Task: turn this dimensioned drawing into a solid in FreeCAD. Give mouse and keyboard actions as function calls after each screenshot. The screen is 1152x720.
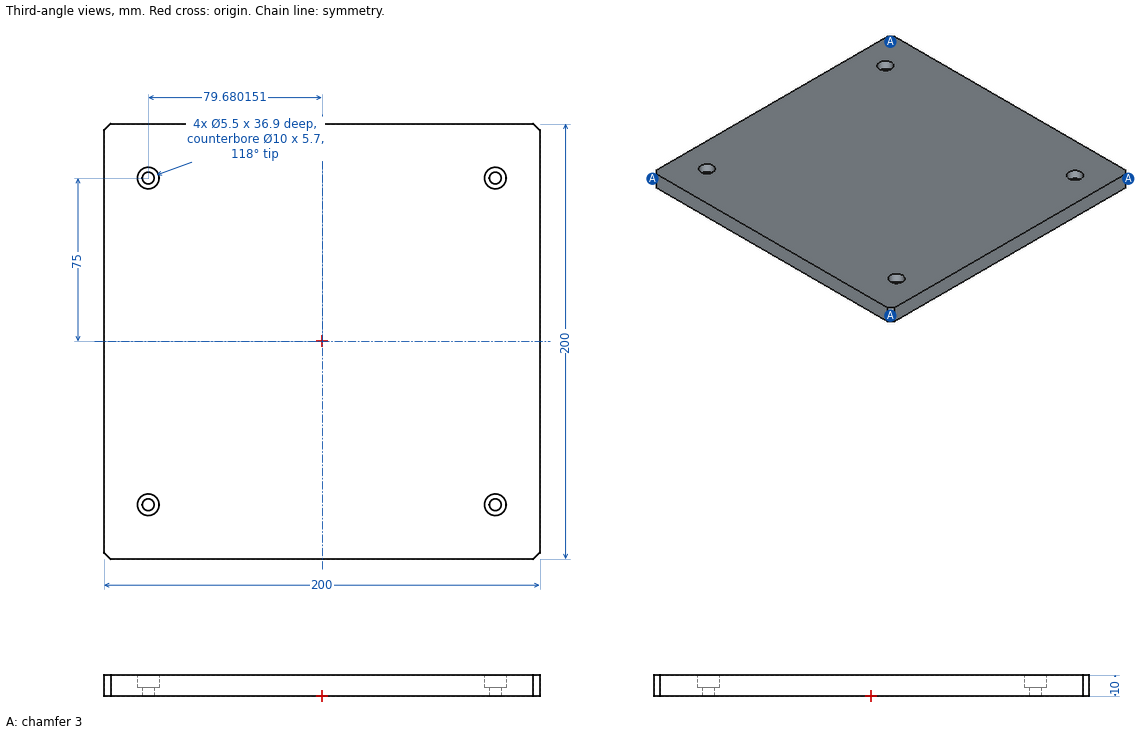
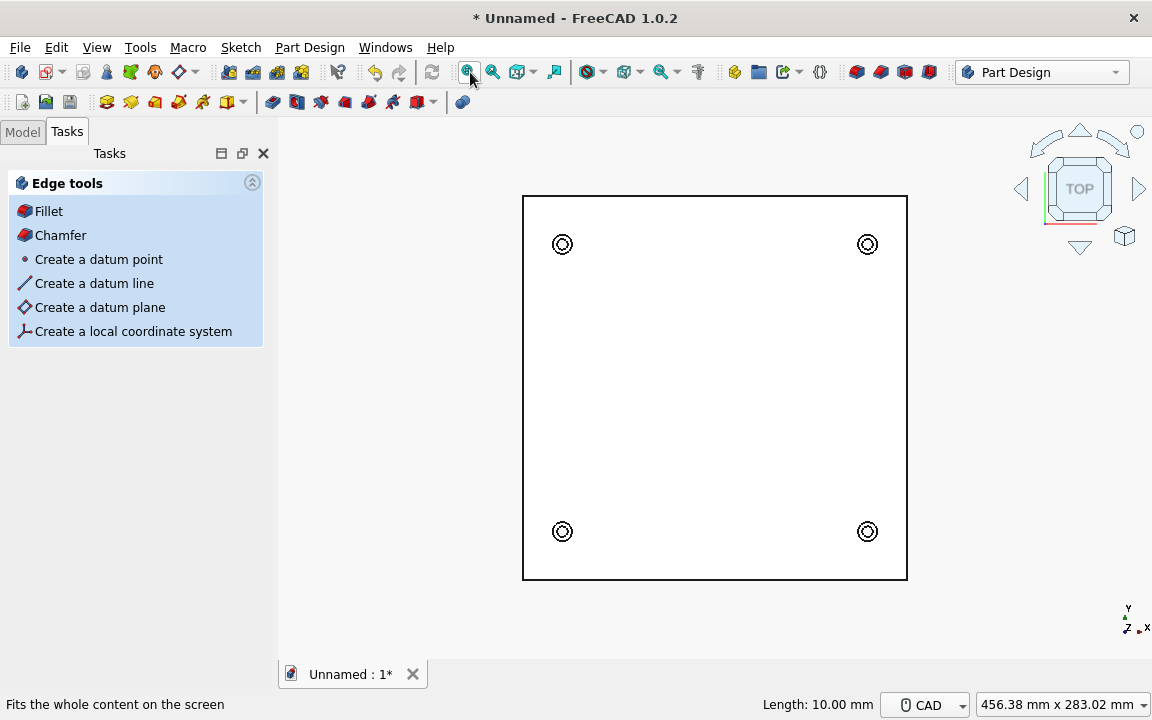
scroll(523, 579, up, 4)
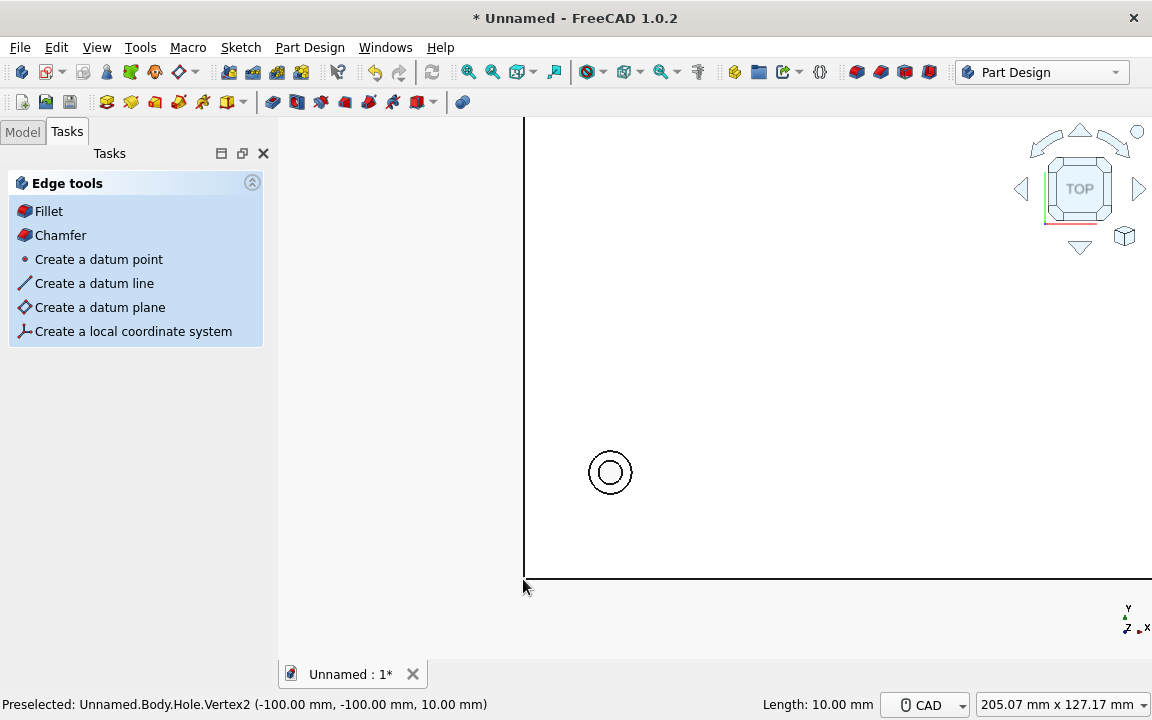
click(470, 72)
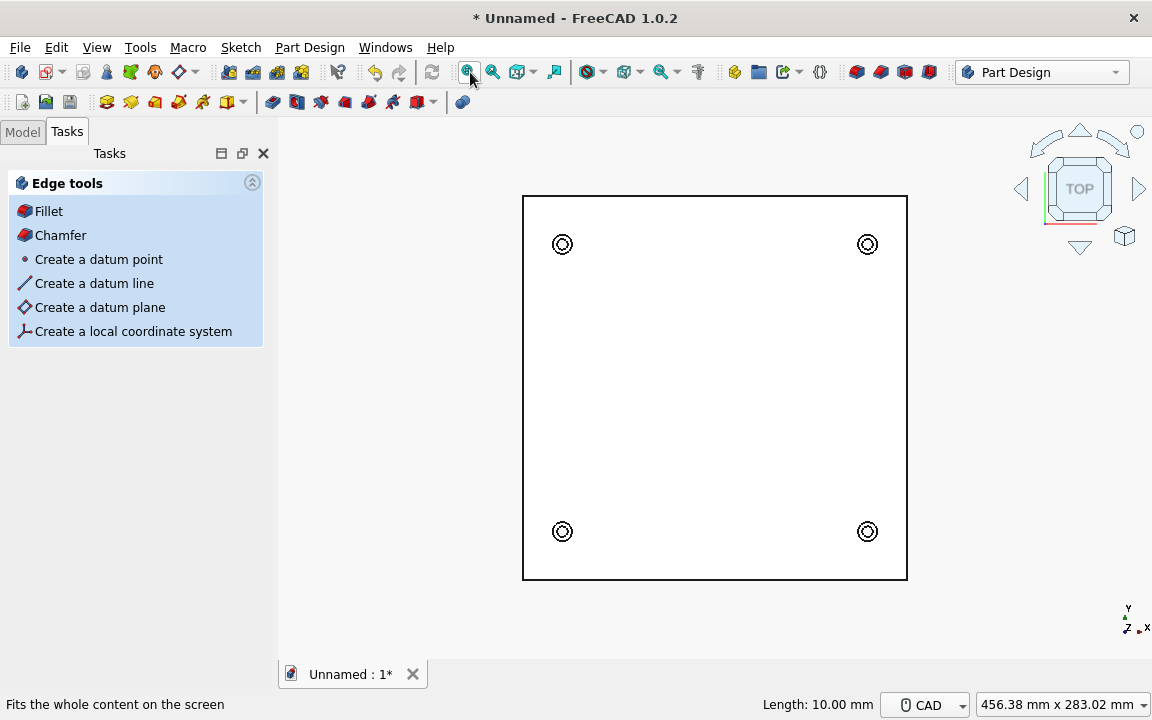
key(1)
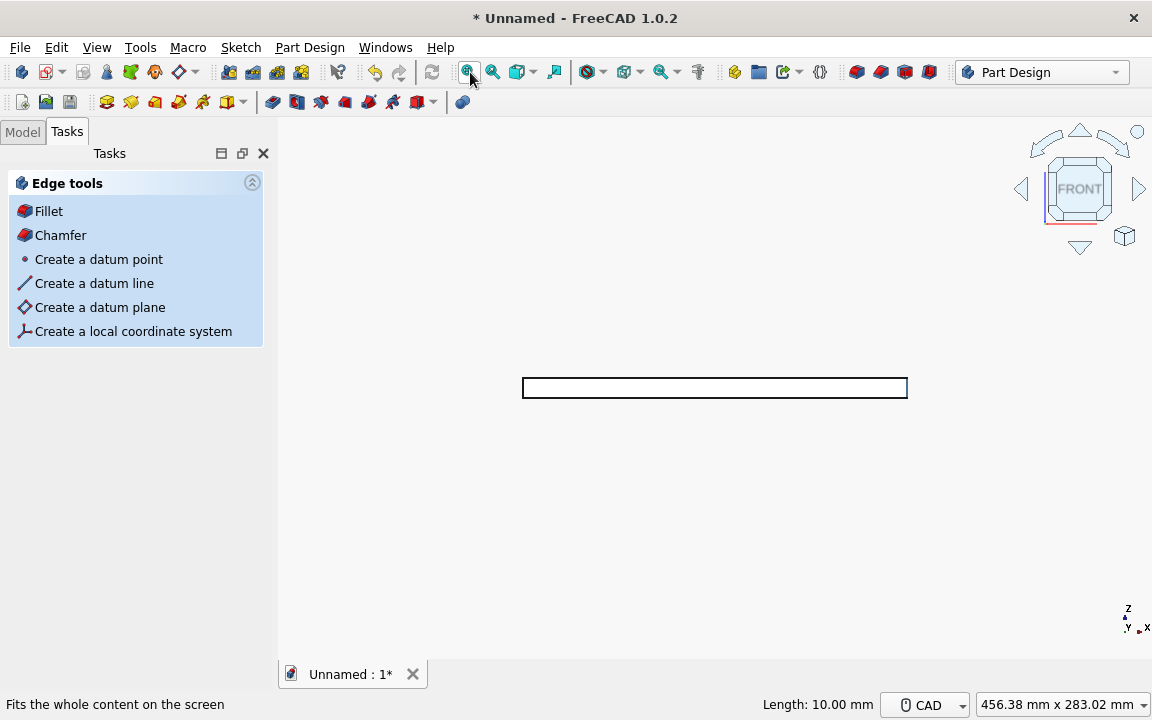
click(470, 72)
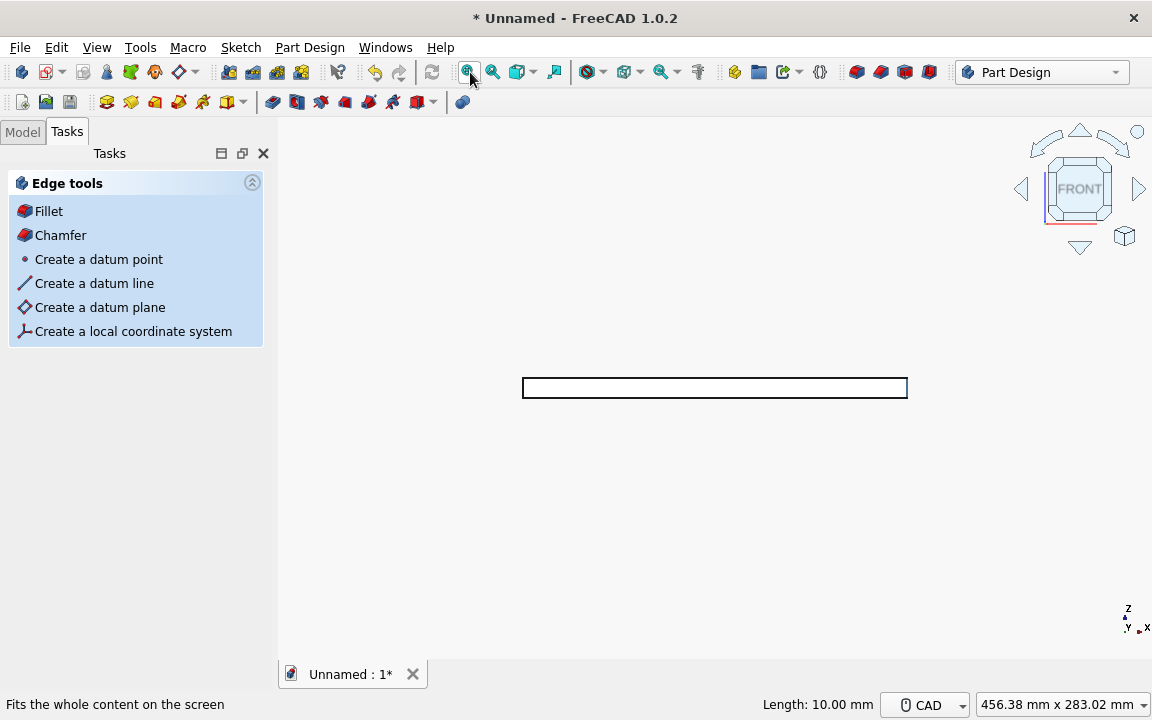
click(523, 387, ctrl)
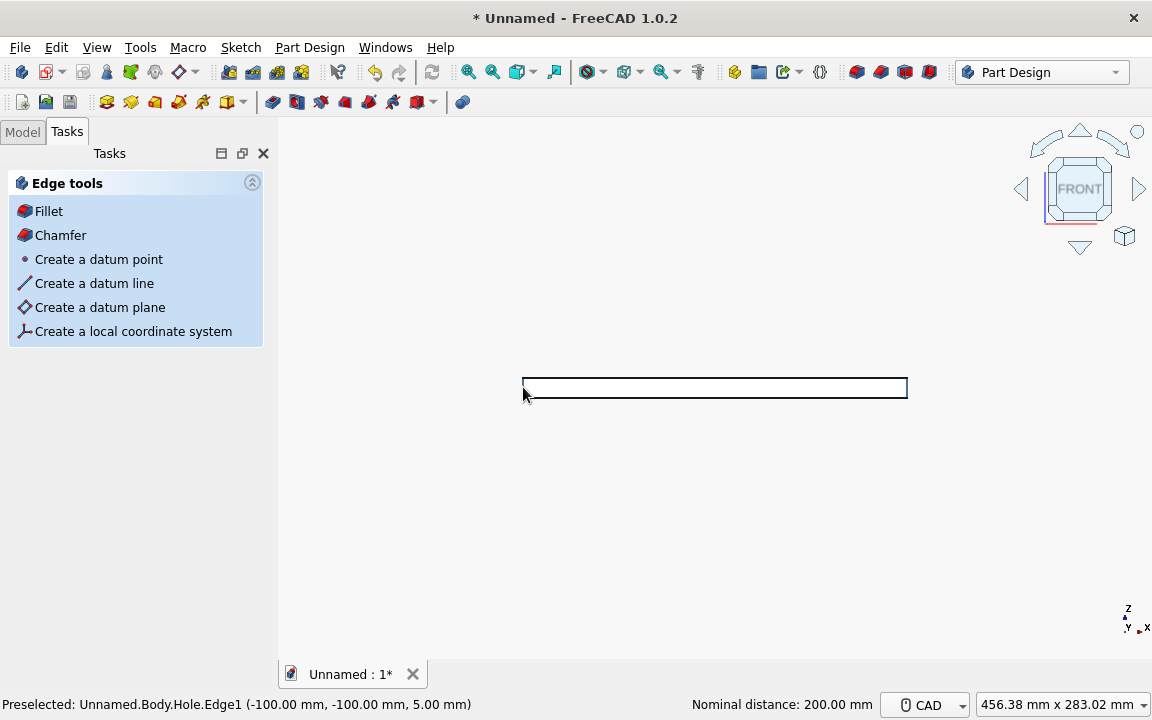
scroll(523, 387, up, 4)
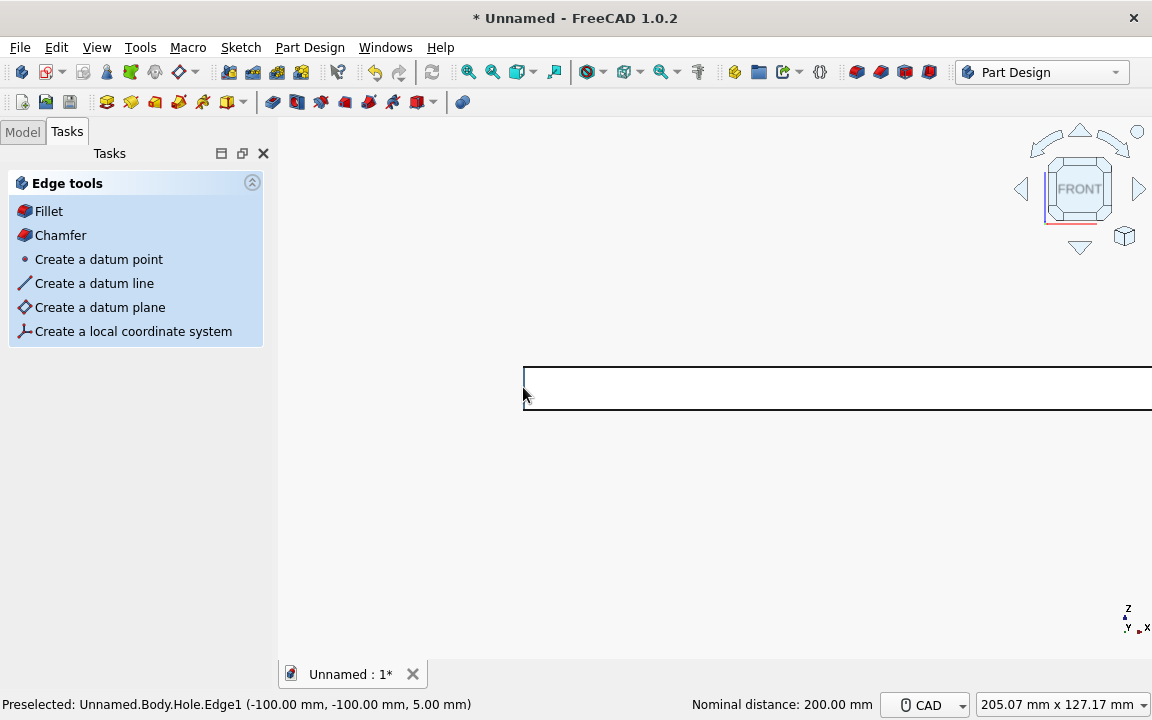
click(470, 72)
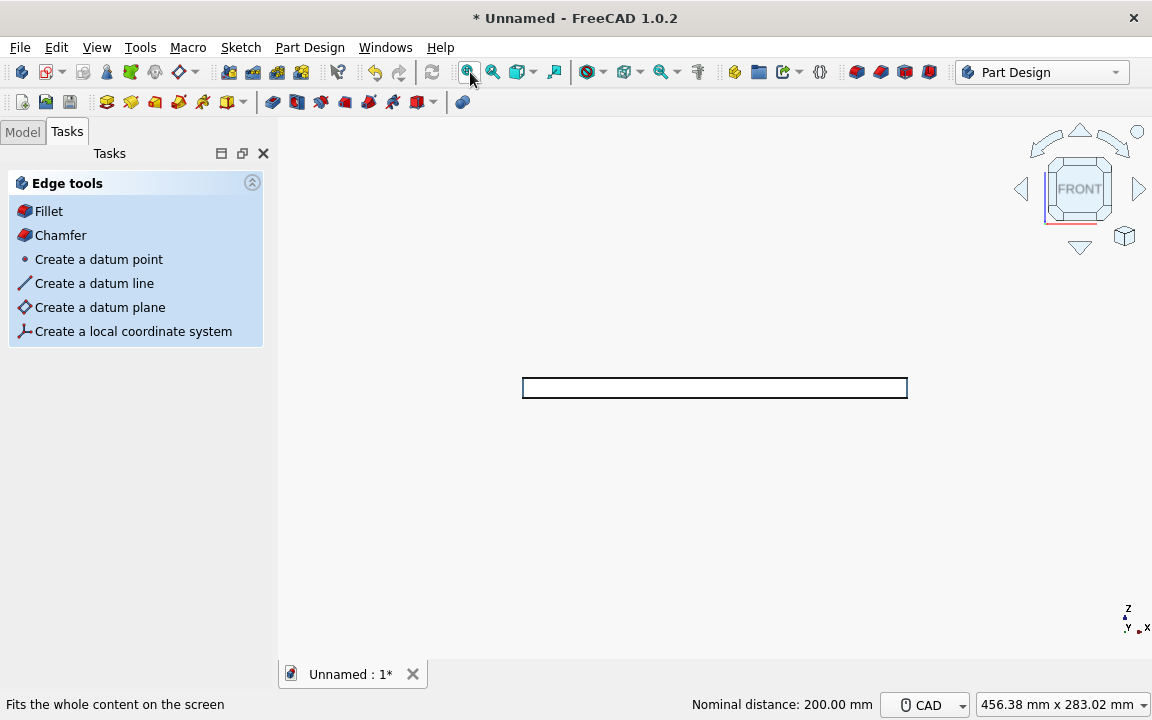
key(3)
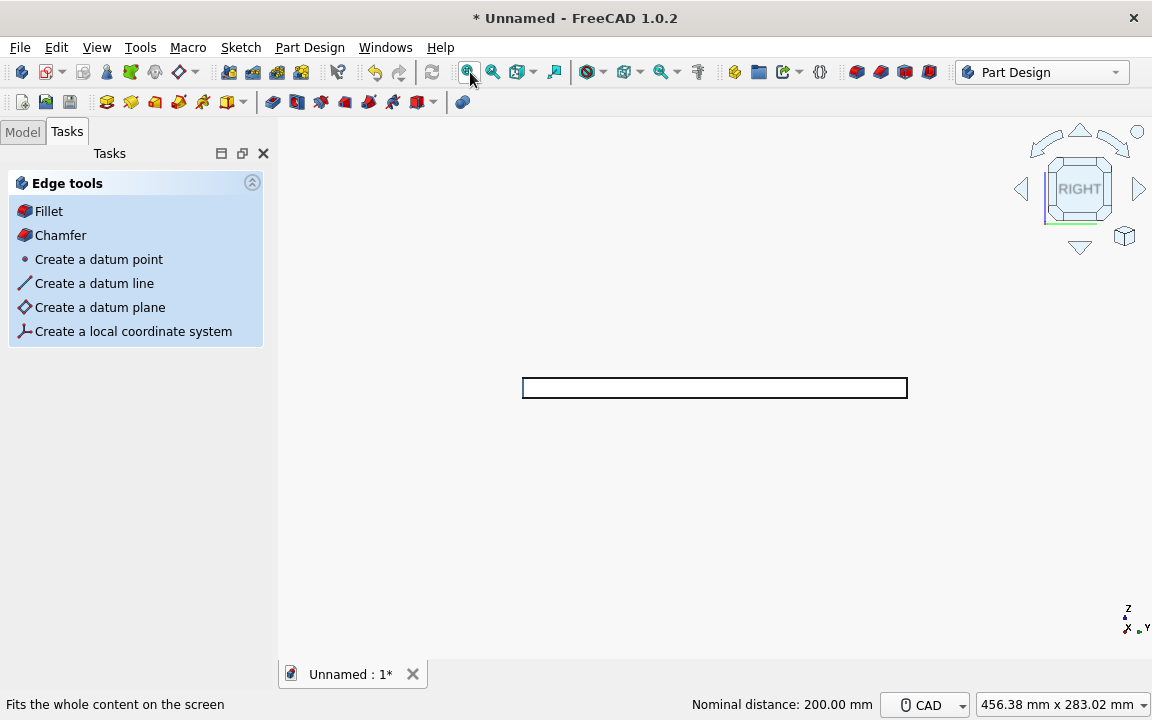
click(470, 72)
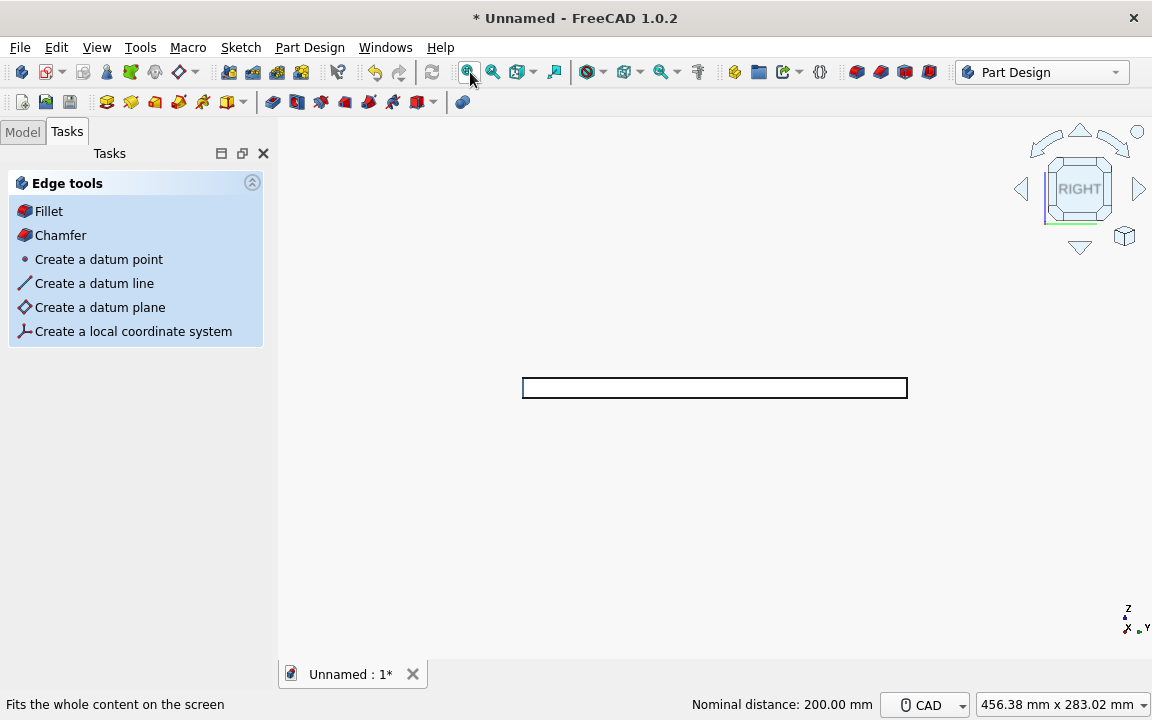
click(907, 387, ctrl)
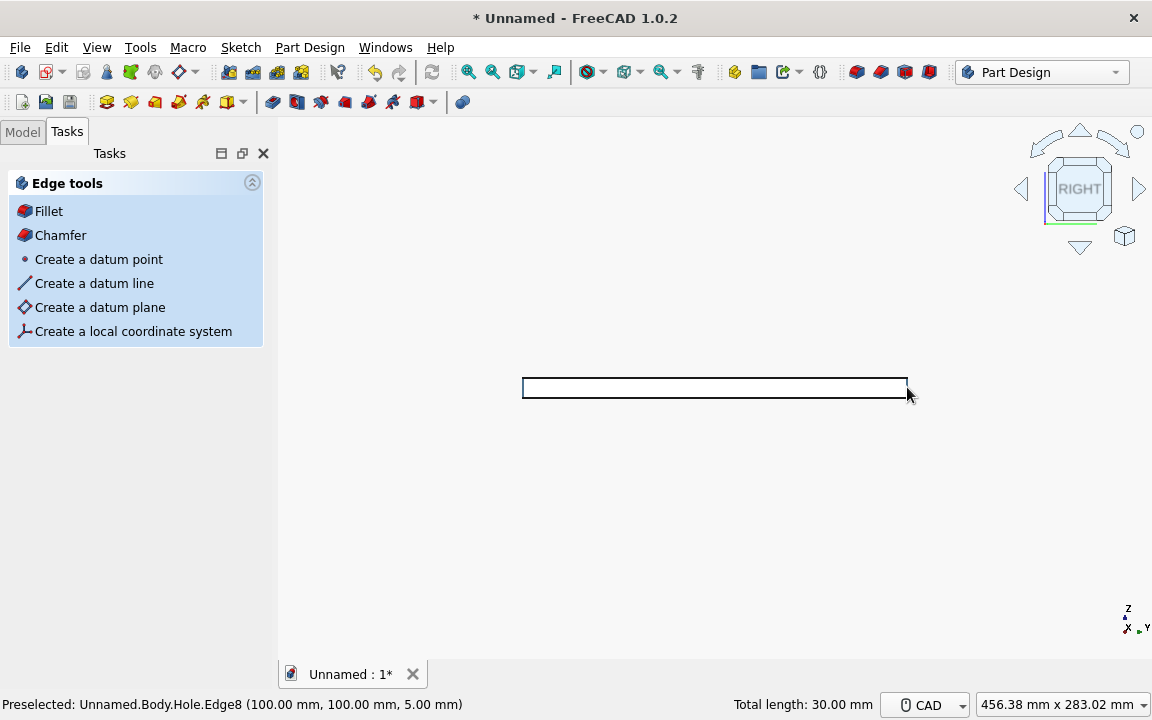
scroll(907, 387, up, 4)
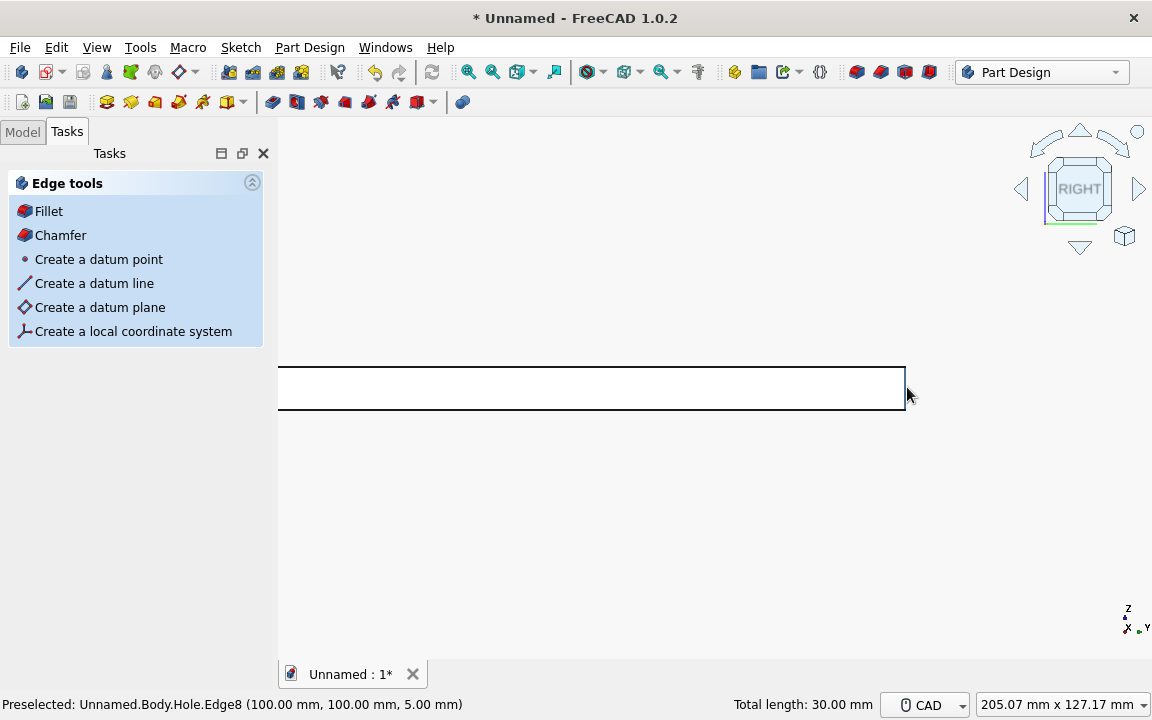
click(470, 72)